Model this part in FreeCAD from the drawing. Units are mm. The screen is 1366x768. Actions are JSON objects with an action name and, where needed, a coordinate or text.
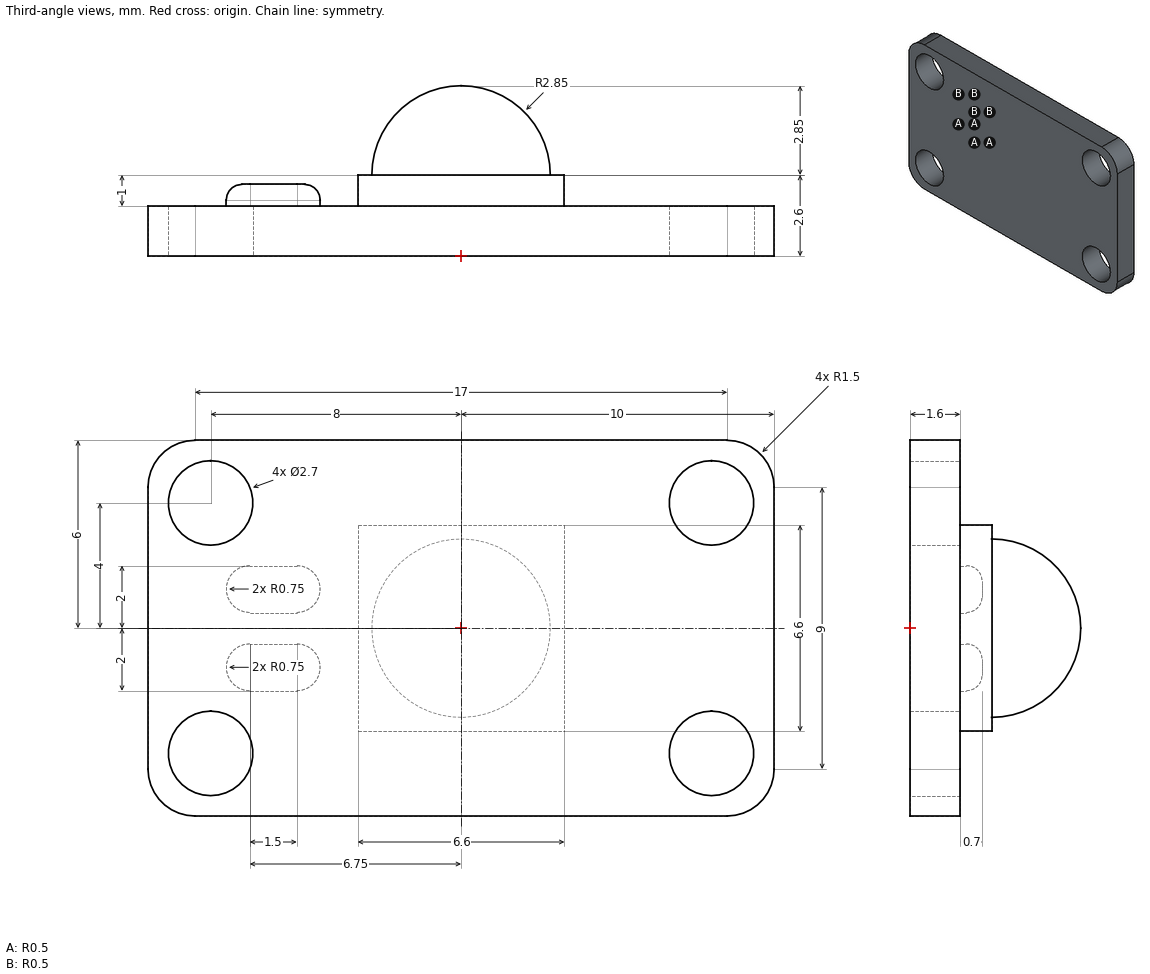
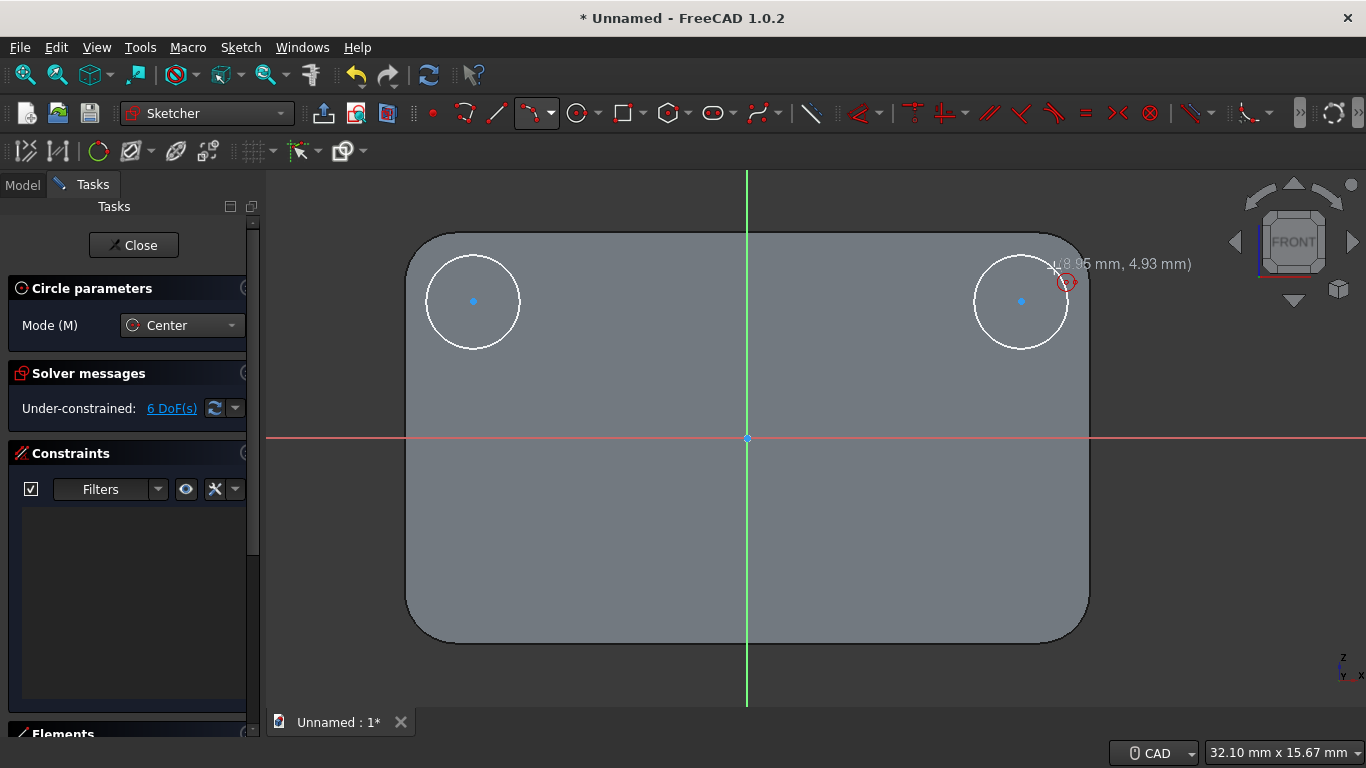
{"action": "left_click", "coordinate": [1021, 575]}
{"action": "left_click", "coordinate": [1054, 542]}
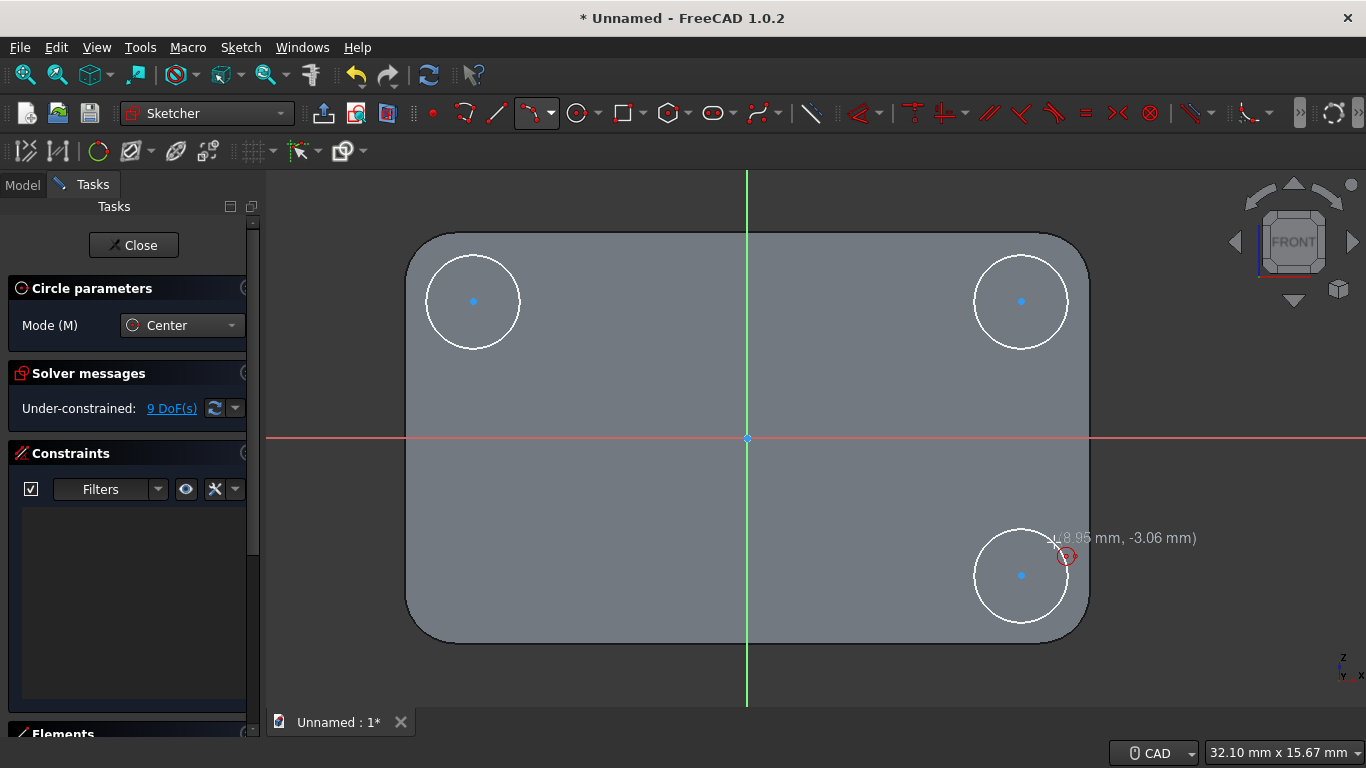
{"action": "left_click", "coordinate": [473, 575]}
{"action": "left_click", "coordinate": [506, 542]}
{"action": "key", "text": "Escape"}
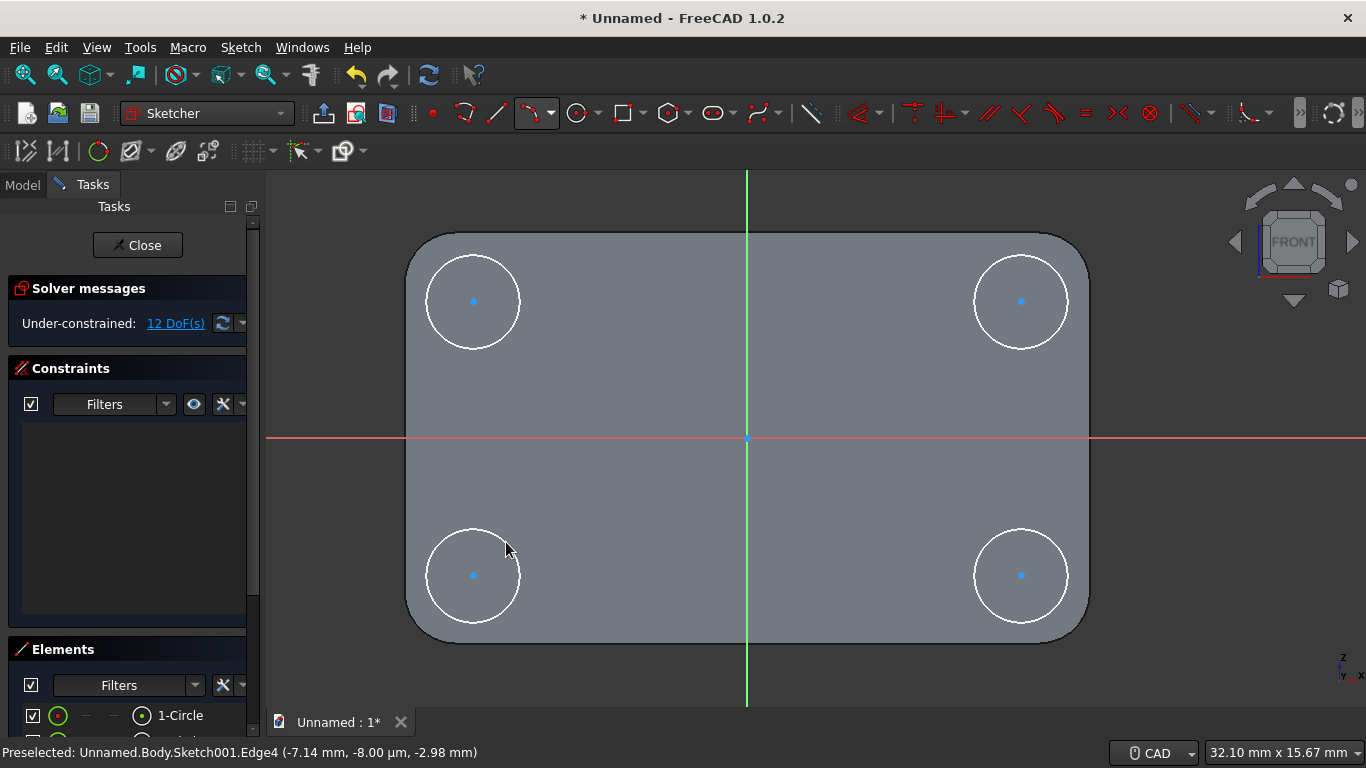
{"action": "left_click", "coordinate": [506, 269]}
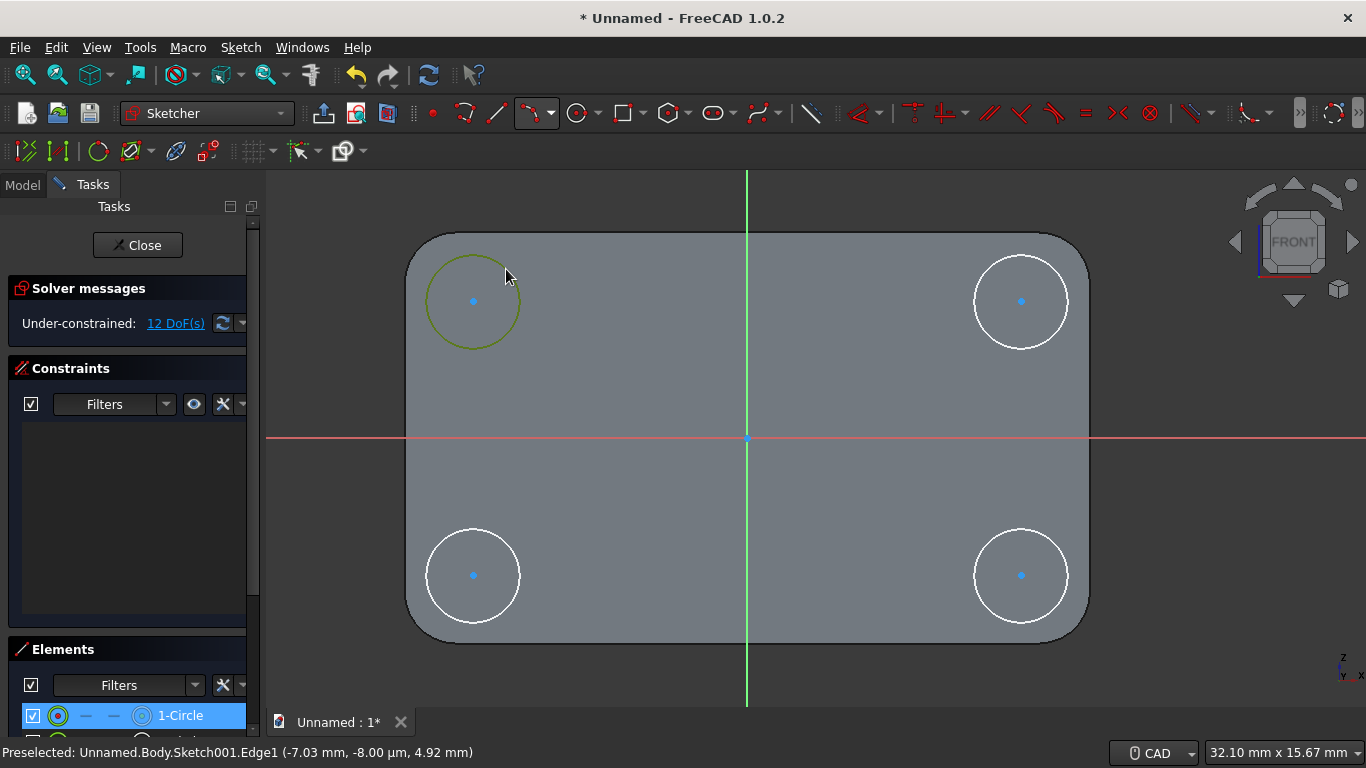
{"action": "left_click", "coordinate": [1054, 269]}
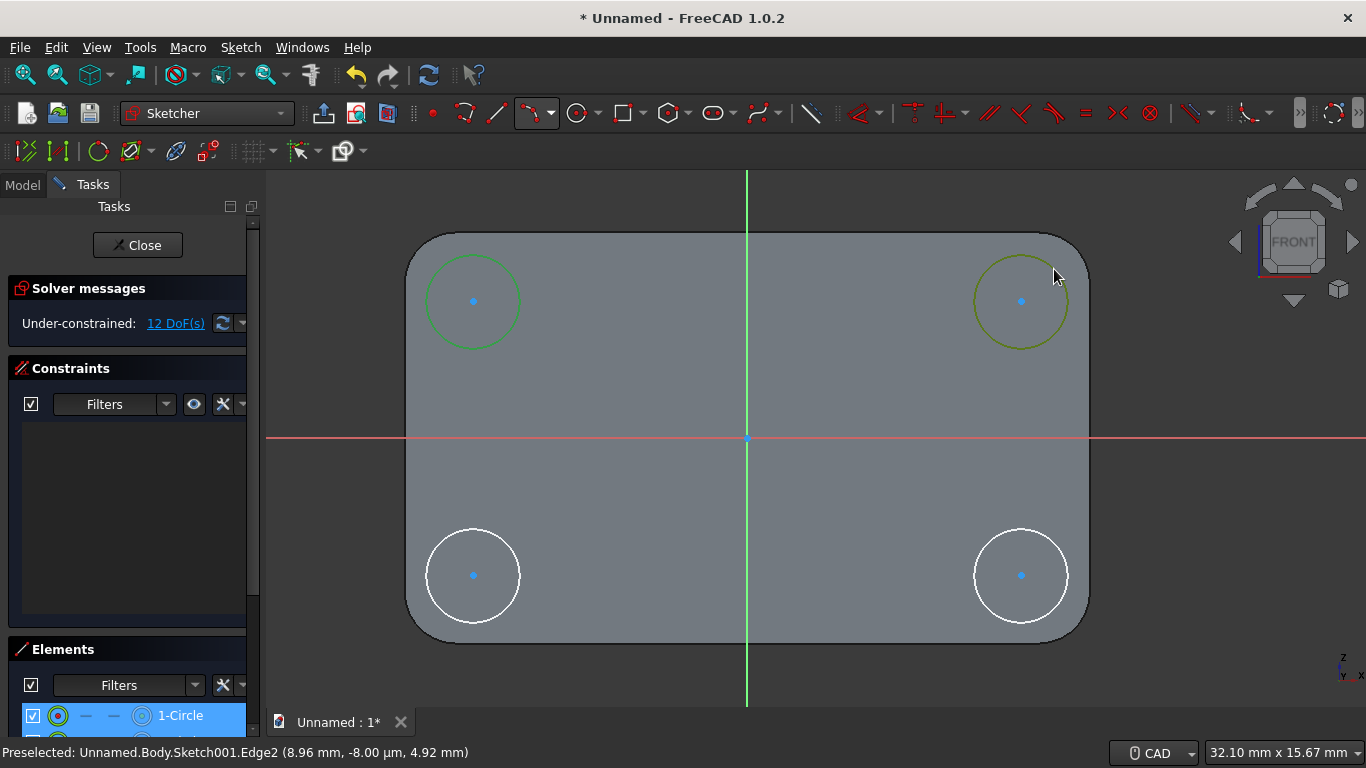
{"action": "left_click", "coordinate": [1054, 543]}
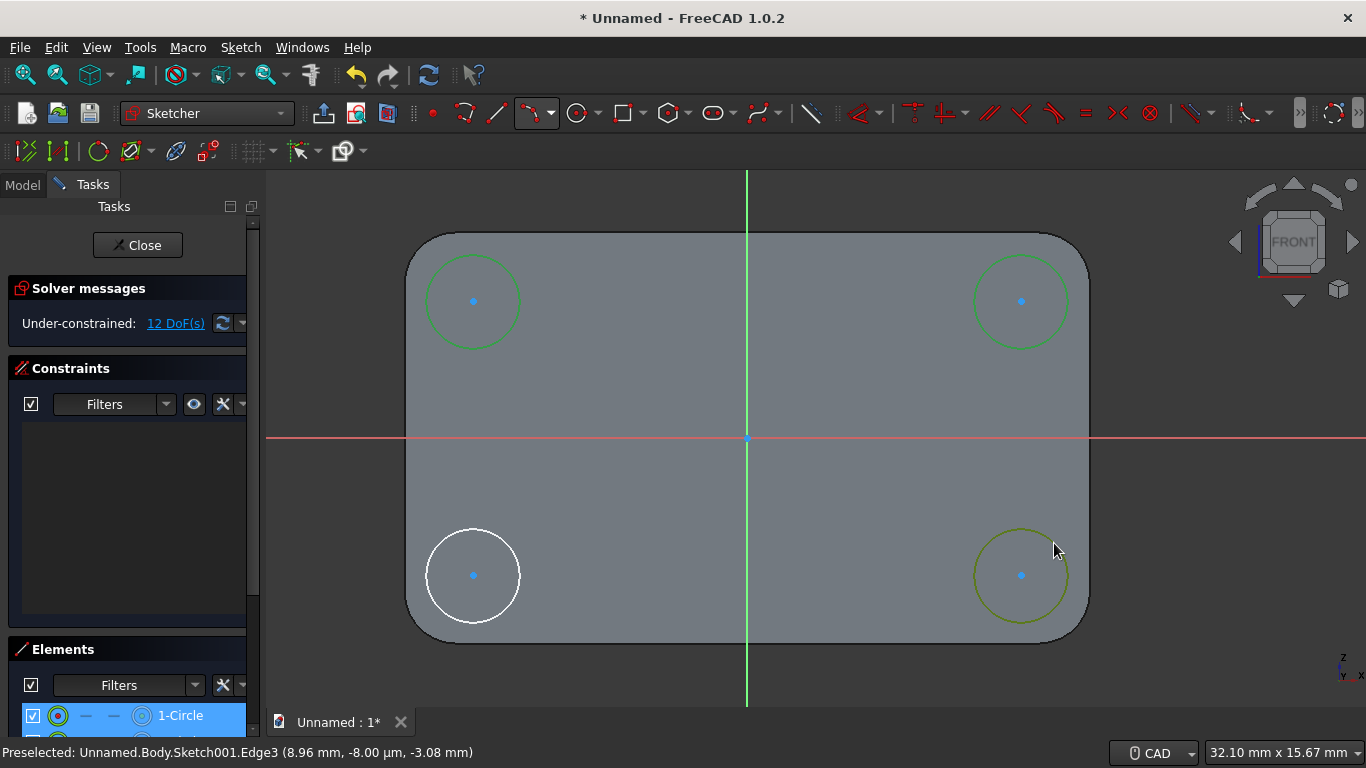
{"action": "left_click", "coordinate": [506, 543]}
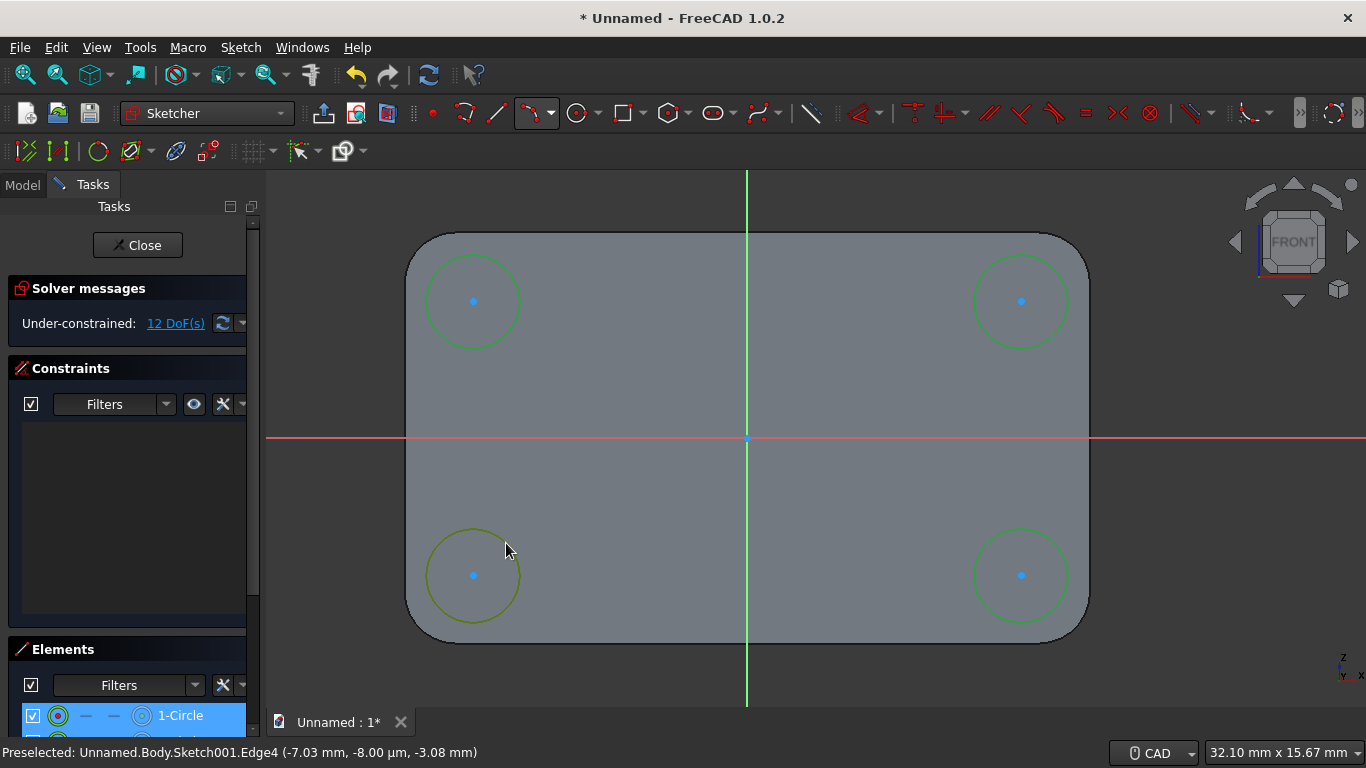
{"action": "left_click", "coordinate": [1086, 114]}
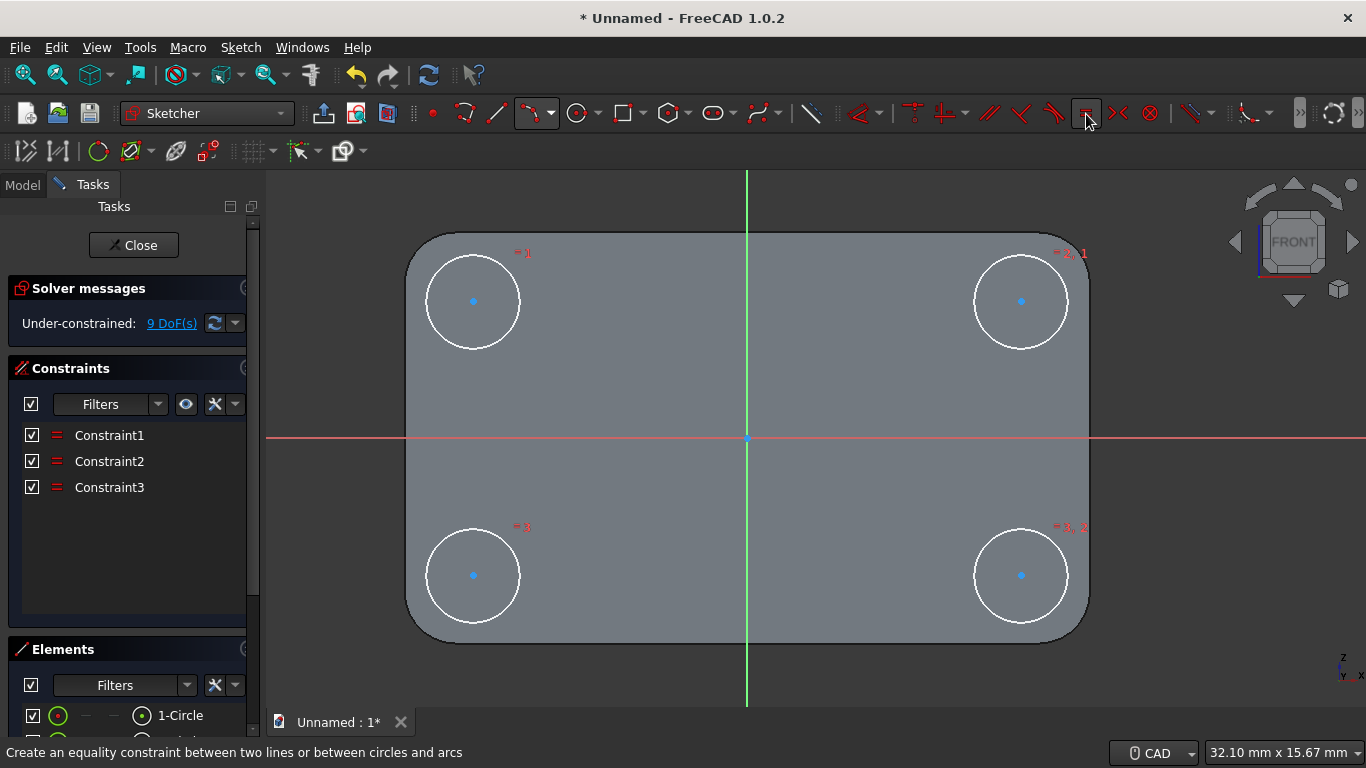
{"action": "left_click", "coordinate": [473, 302]}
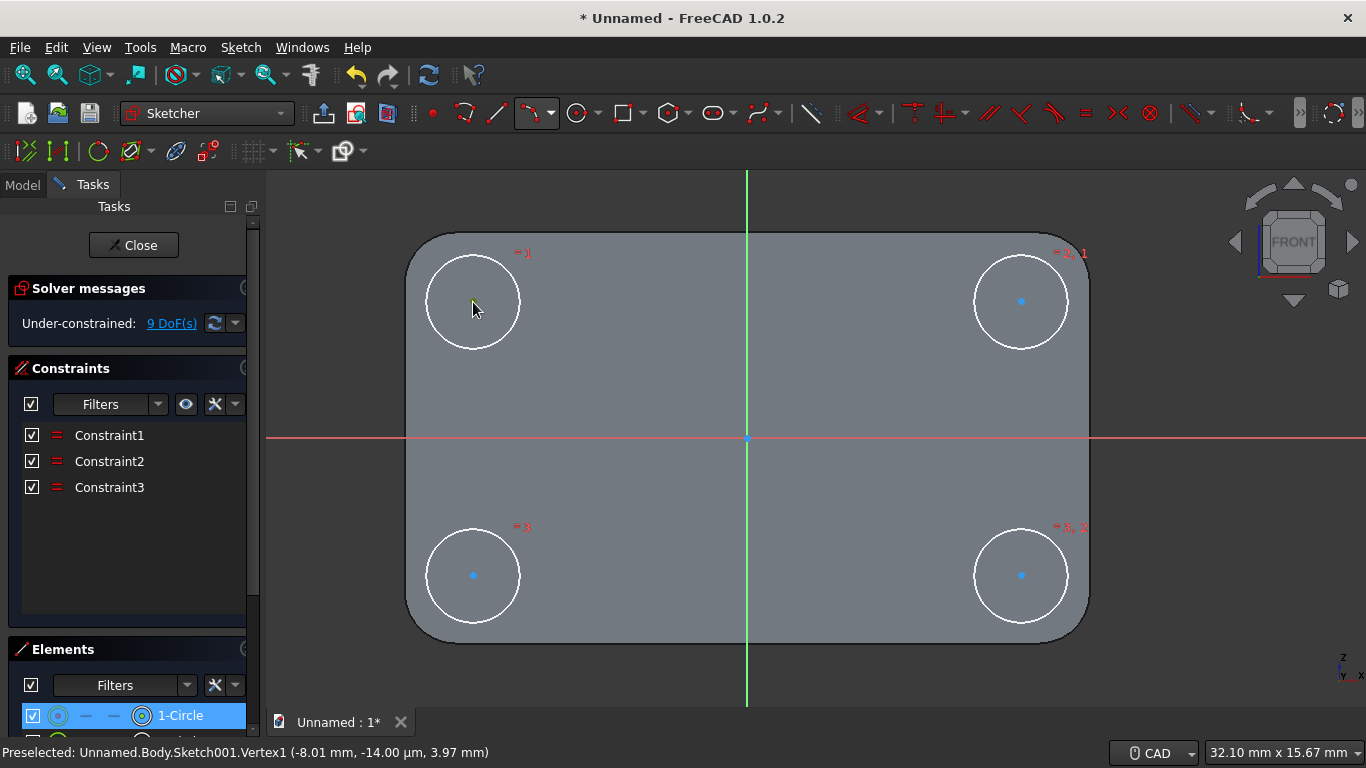
{"action": "left_click", "coordinate": [1021, 302]}